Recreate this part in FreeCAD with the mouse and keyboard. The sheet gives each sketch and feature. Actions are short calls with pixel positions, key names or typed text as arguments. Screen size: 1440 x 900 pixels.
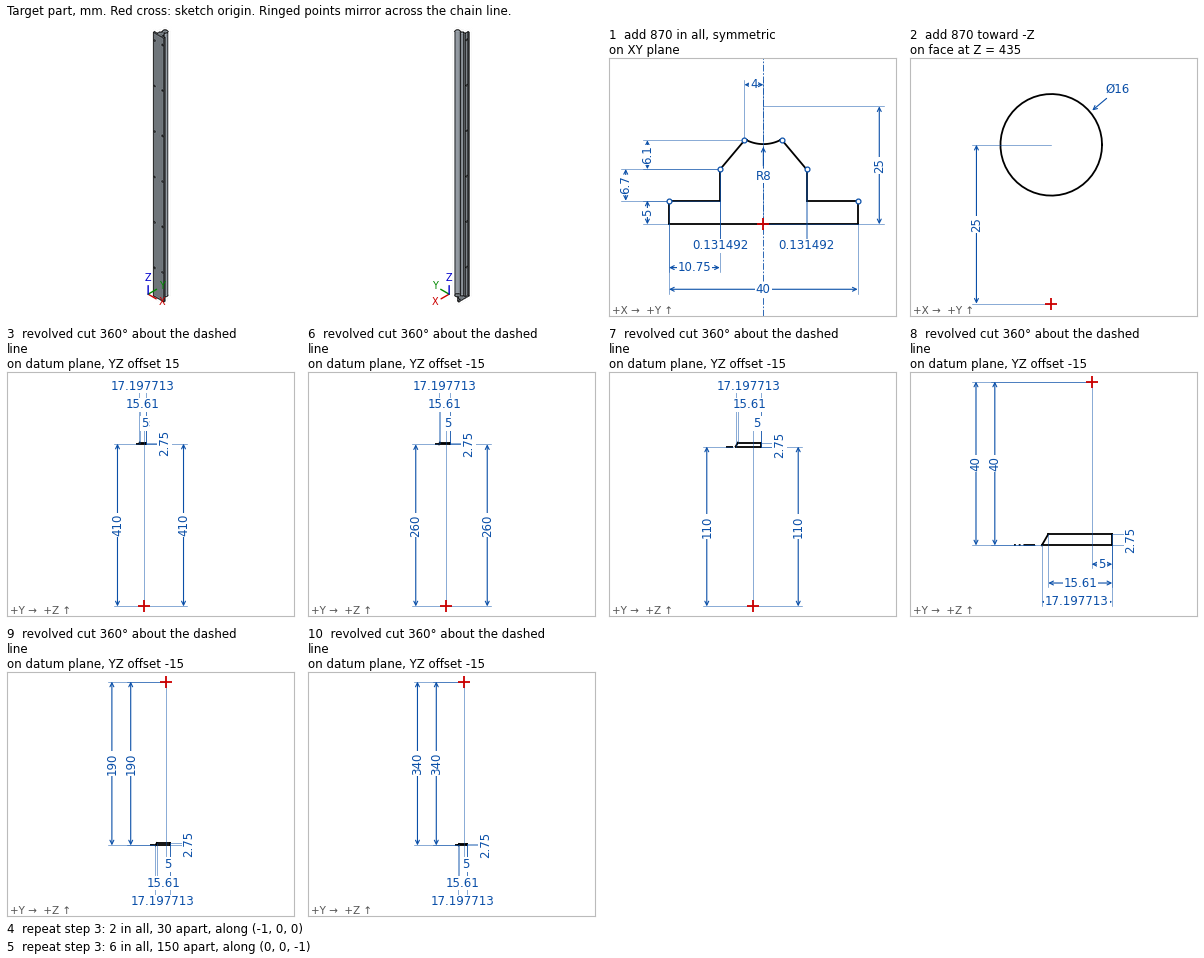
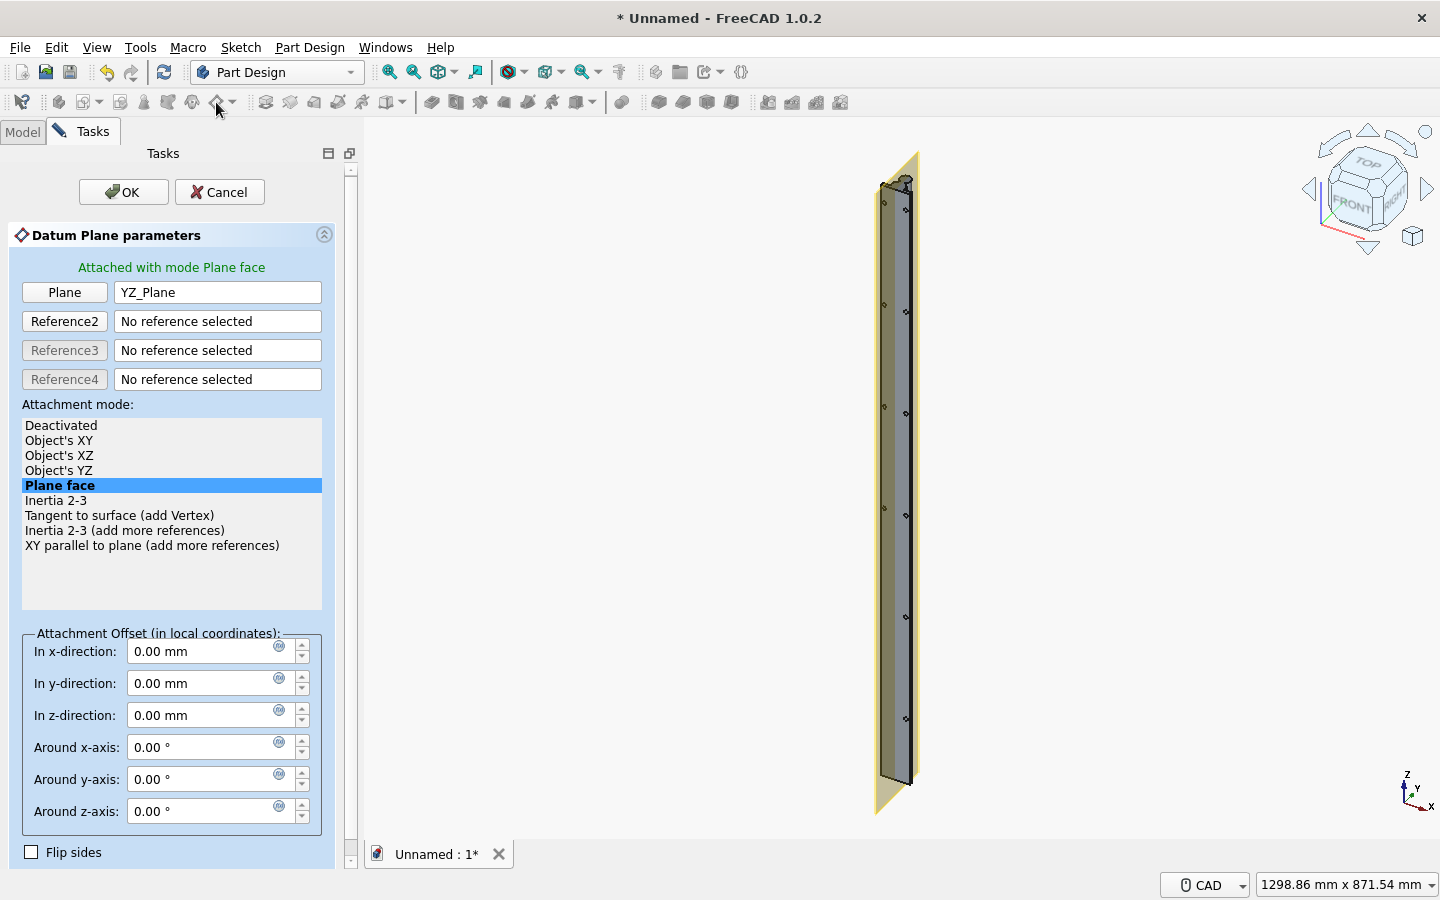
triple_click(210, 715)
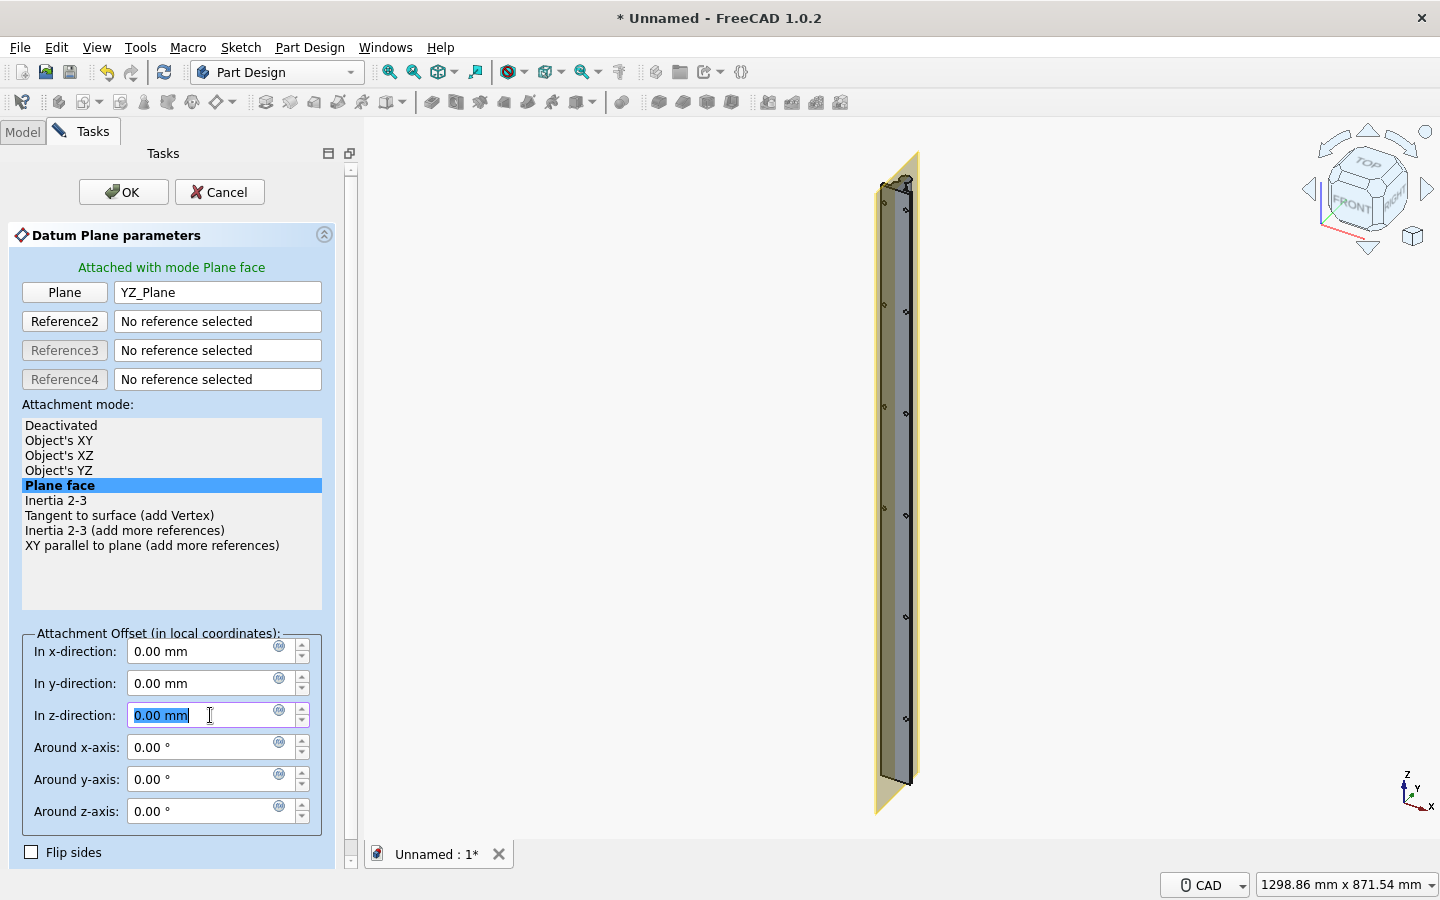
text(-15)
key(Tab)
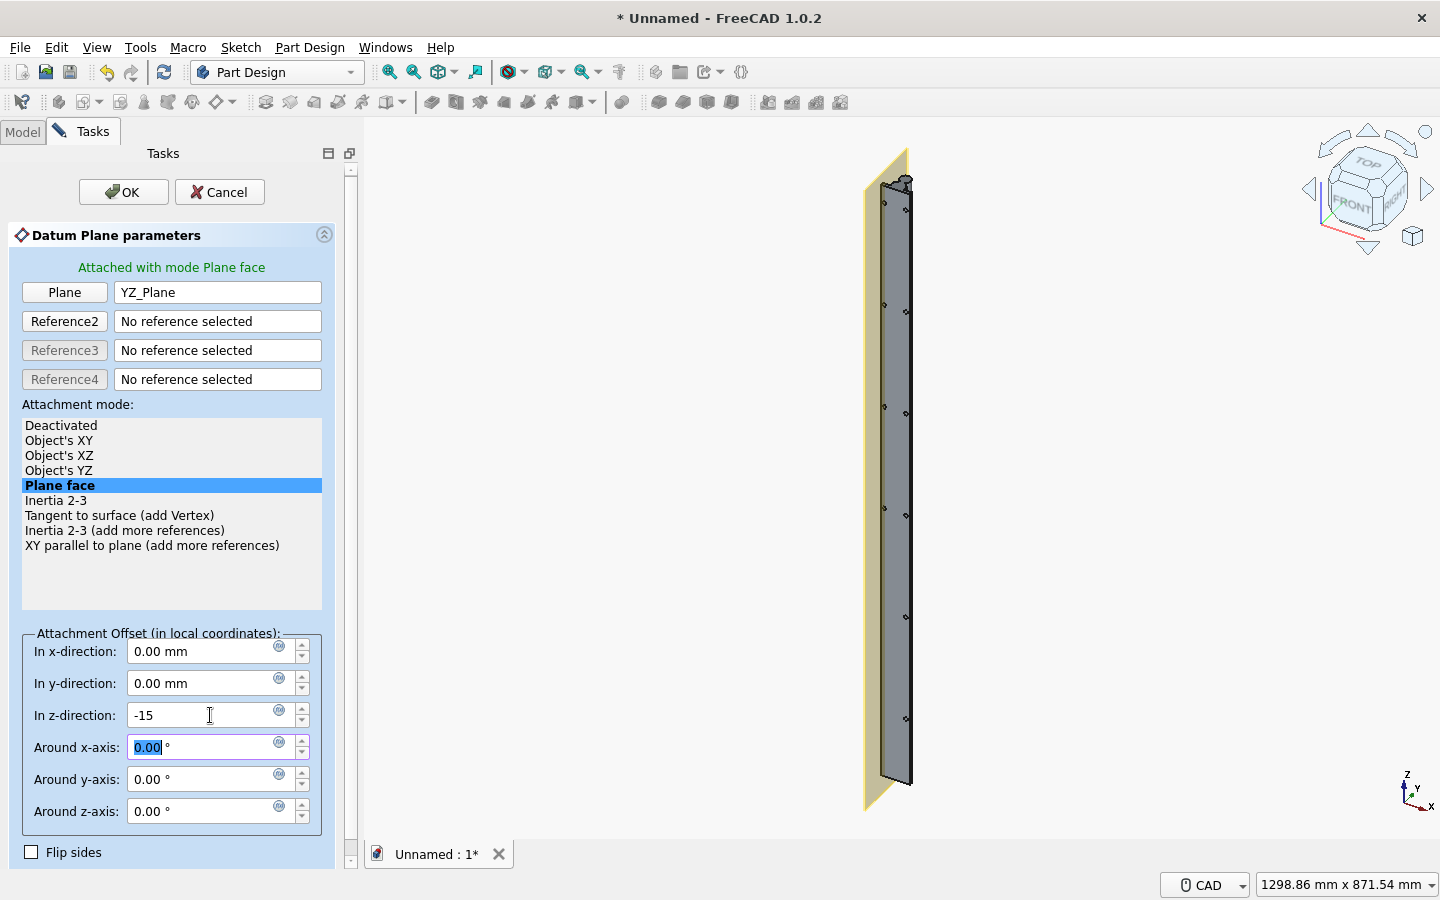
click(124, 192)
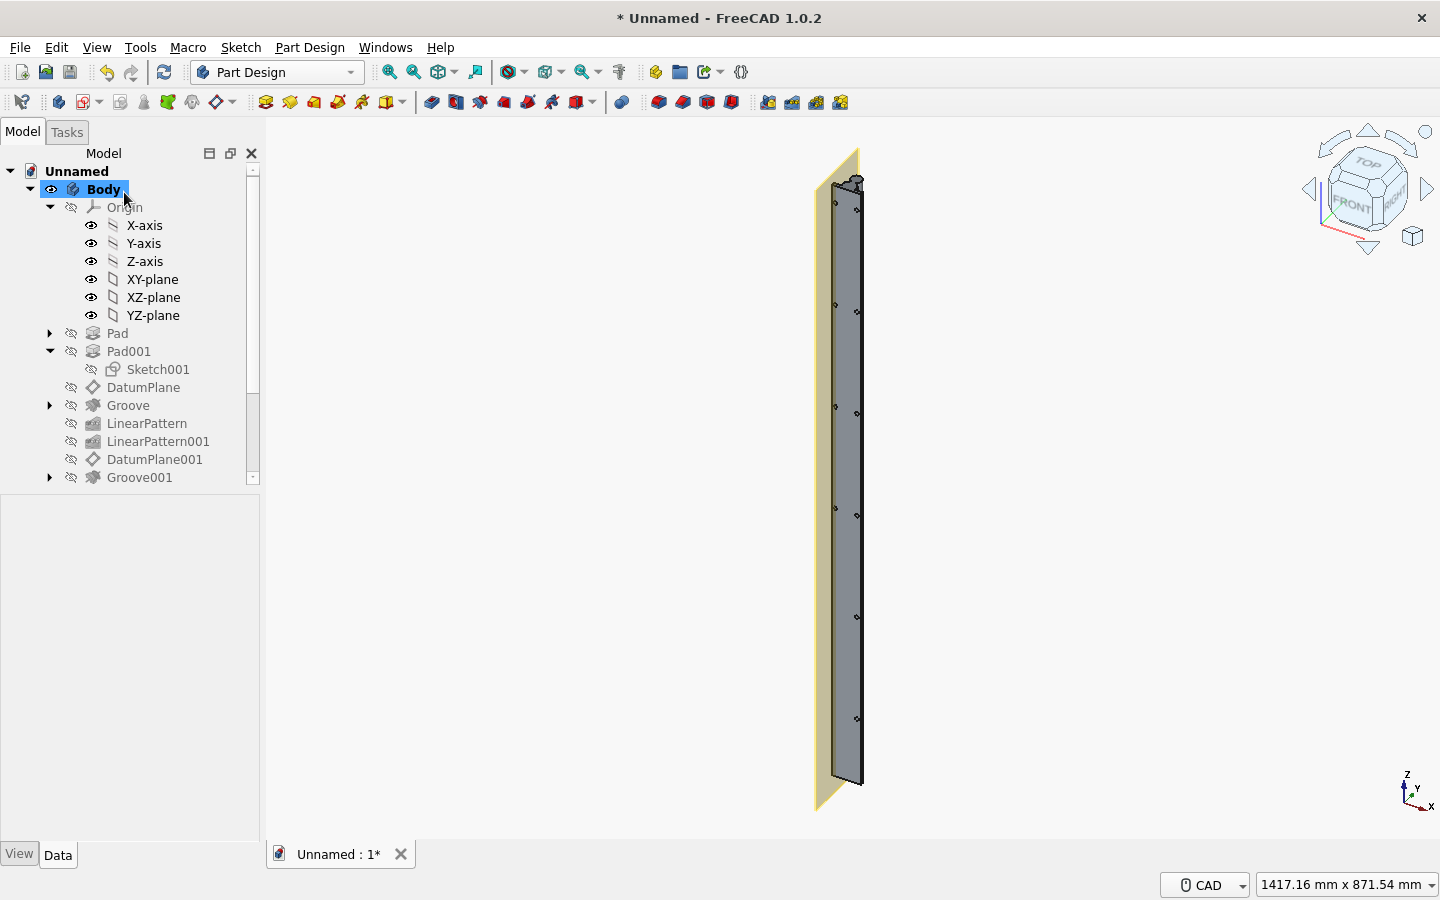
scroll(100, 329, down, 3)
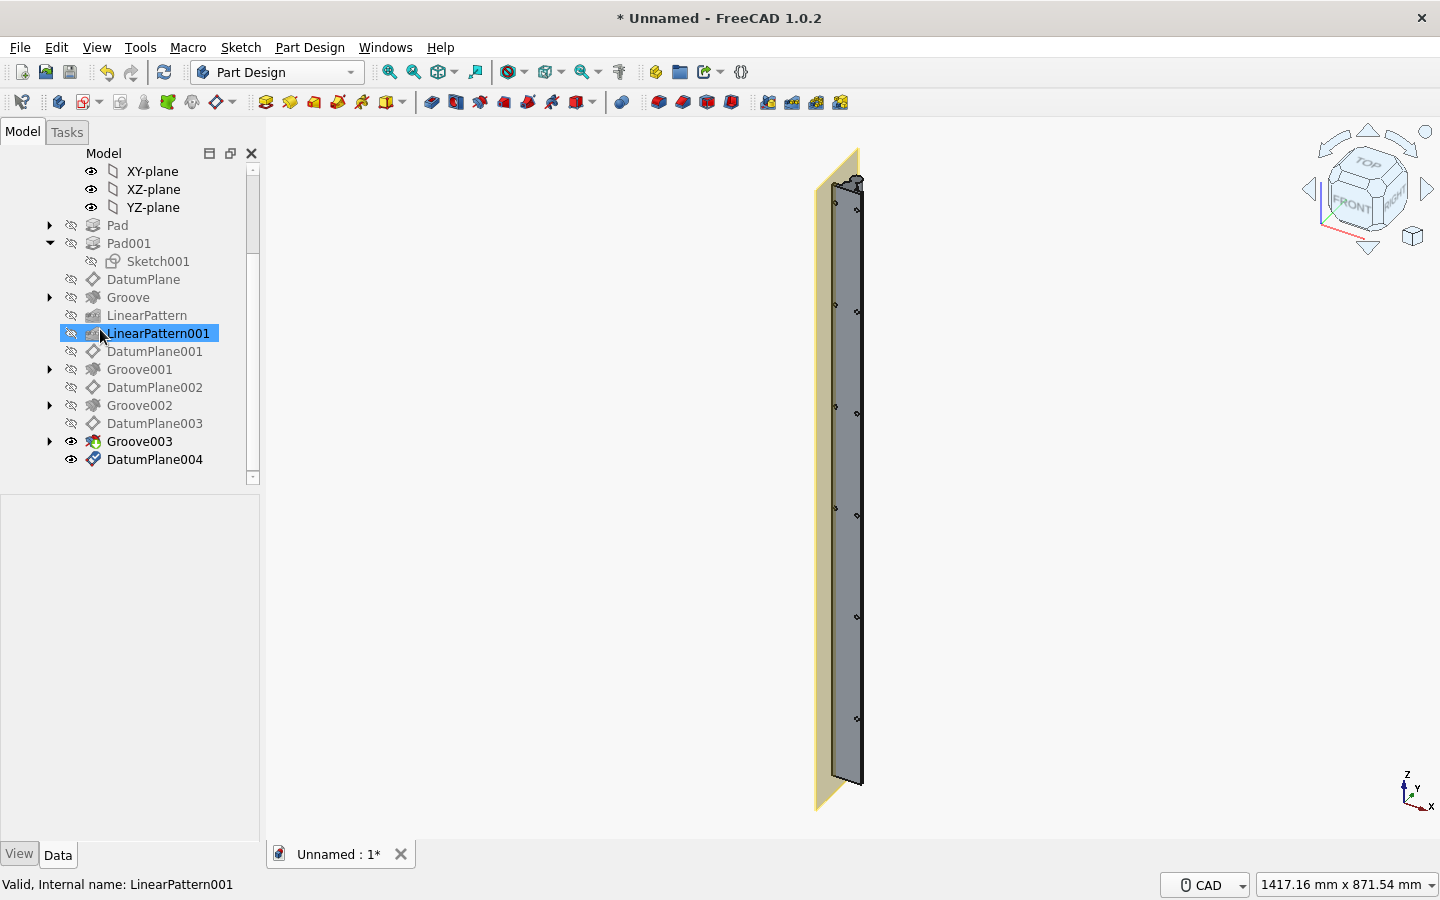
click(116, 459)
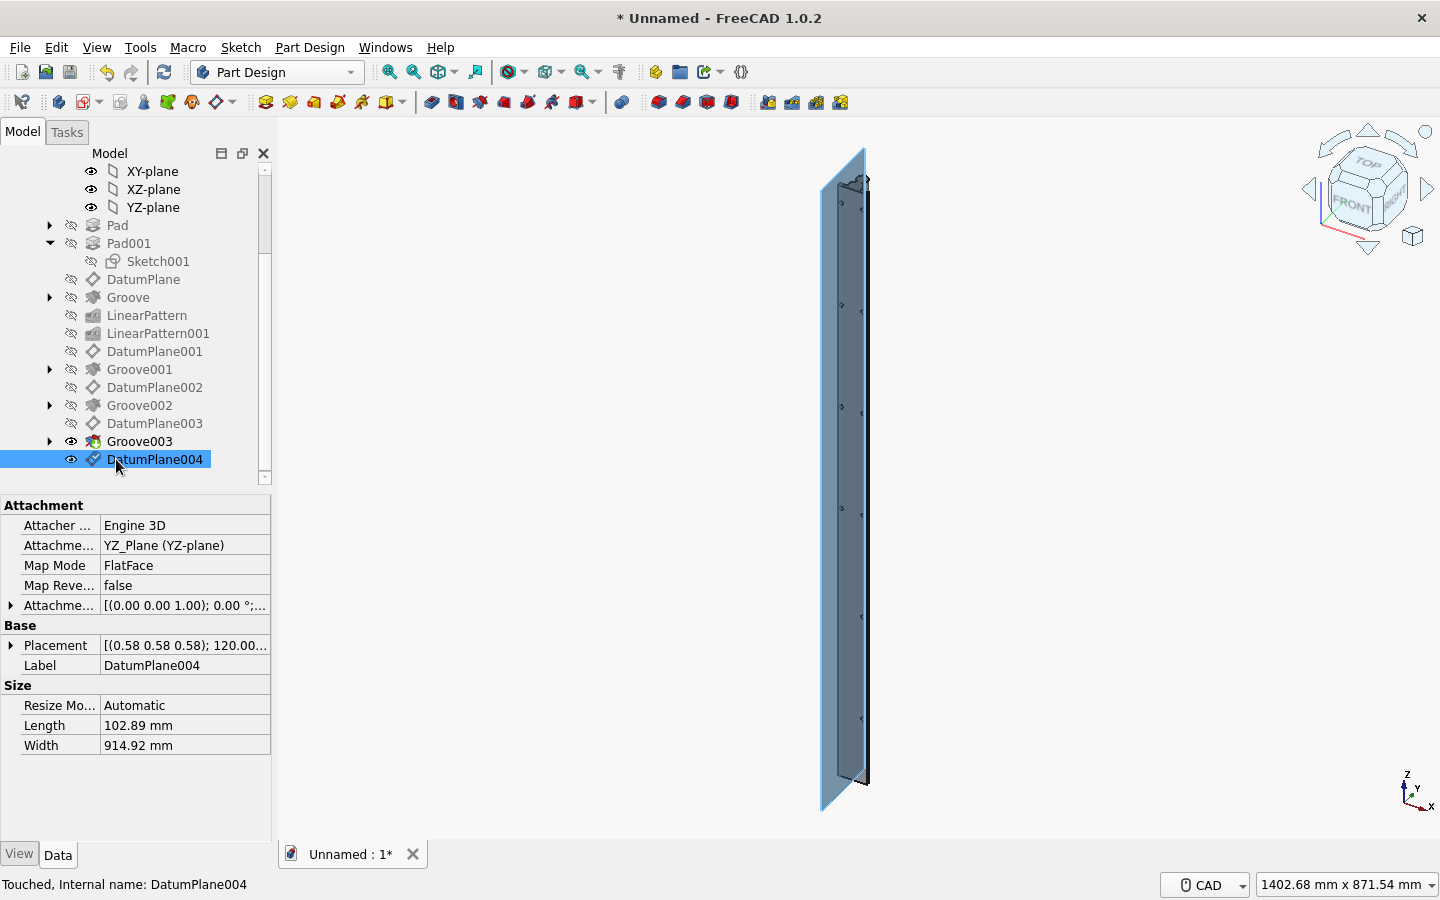
click(84, 102)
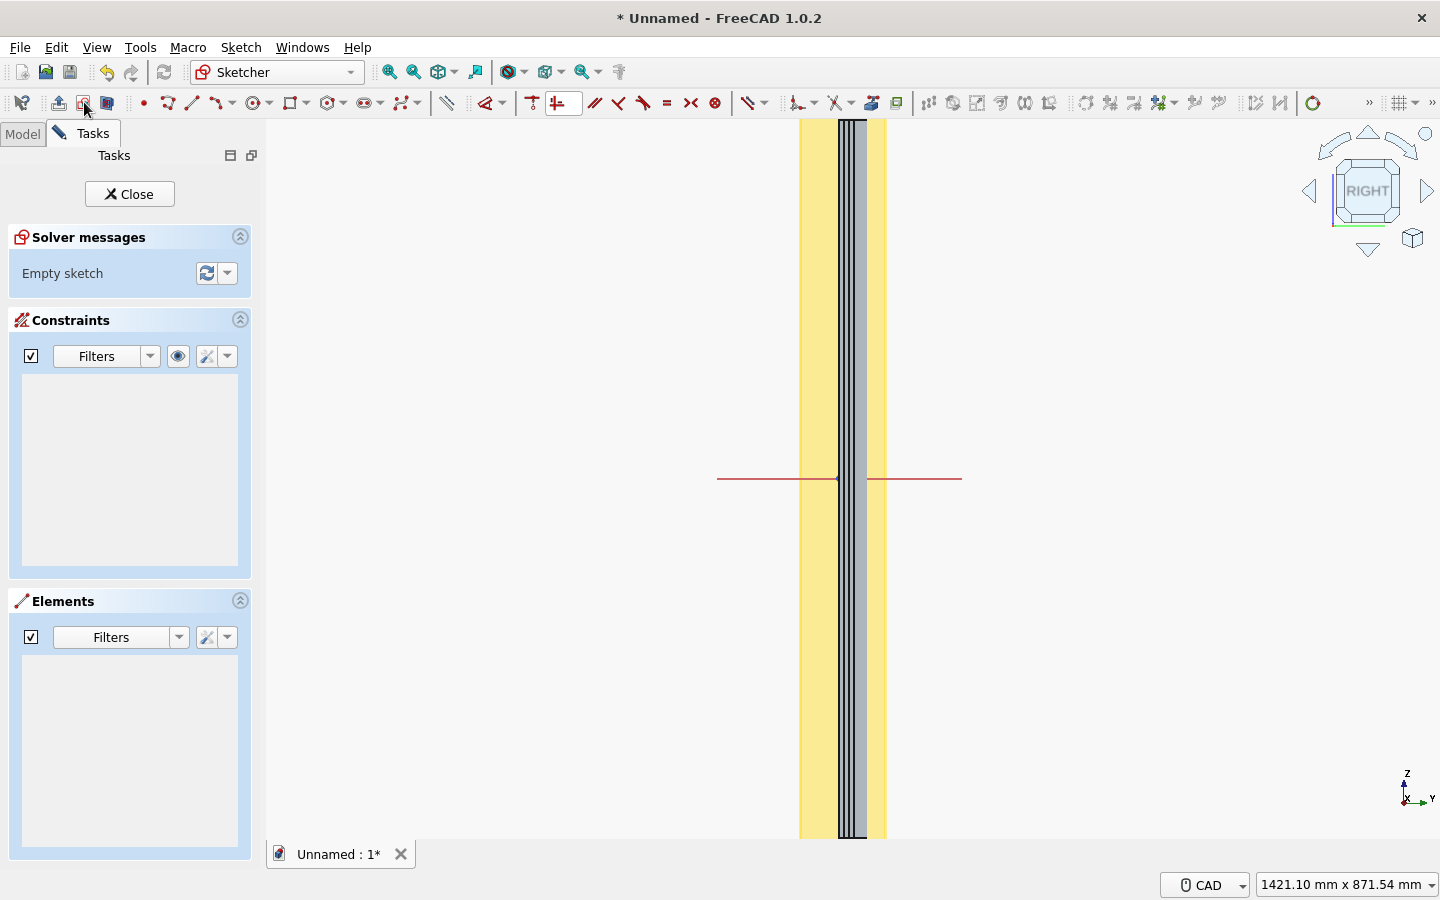
click(108, 104)